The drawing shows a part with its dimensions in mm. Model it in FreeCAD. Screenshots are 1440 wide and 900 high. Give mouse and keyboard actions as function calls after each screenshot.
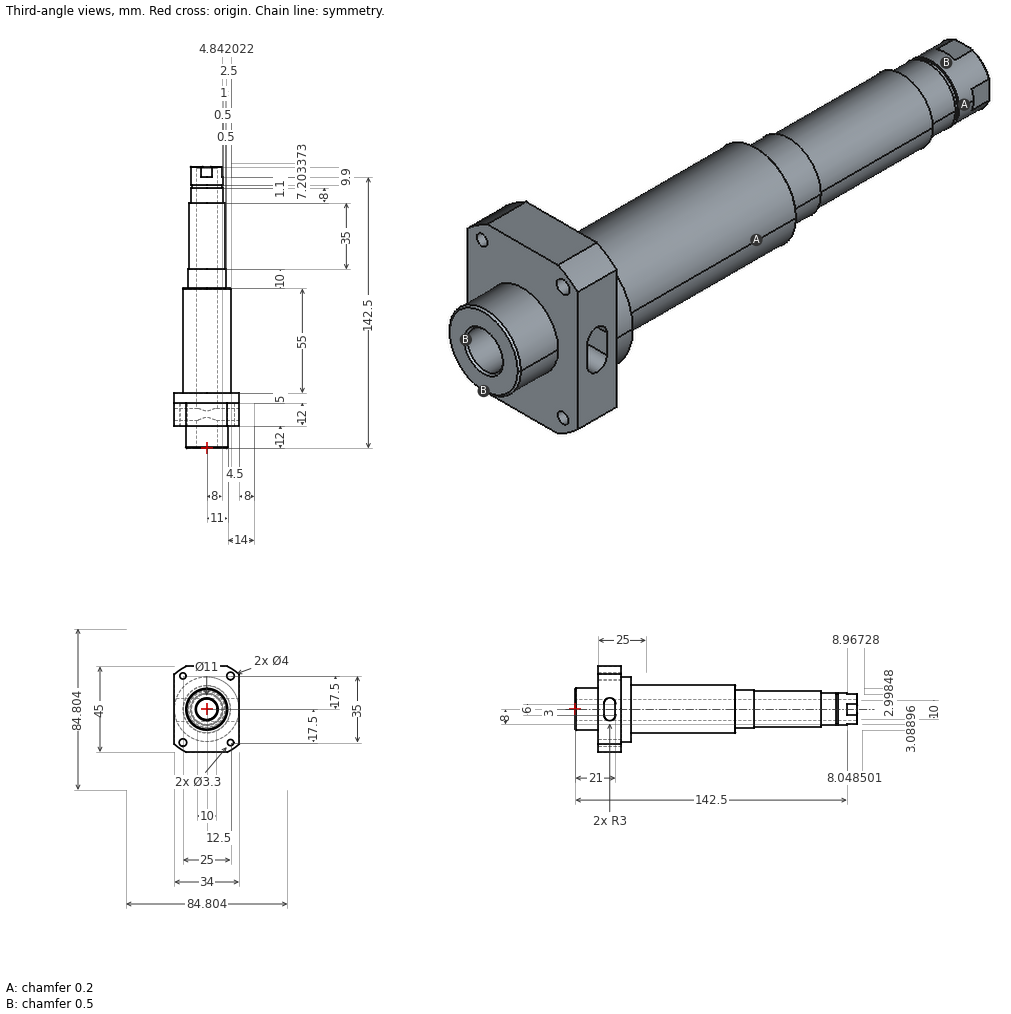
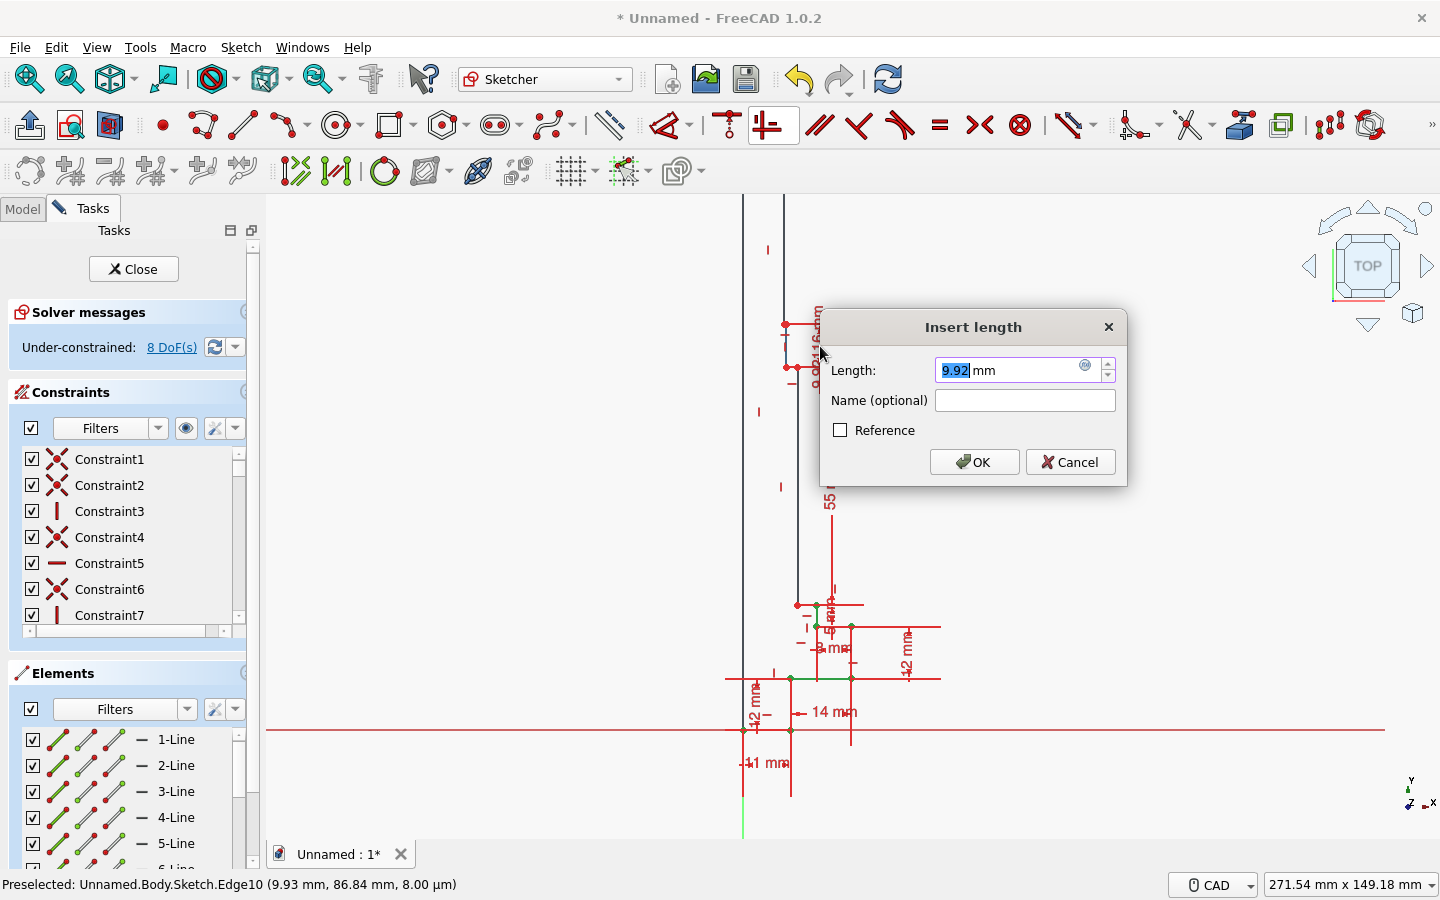
text(10)
key(Return)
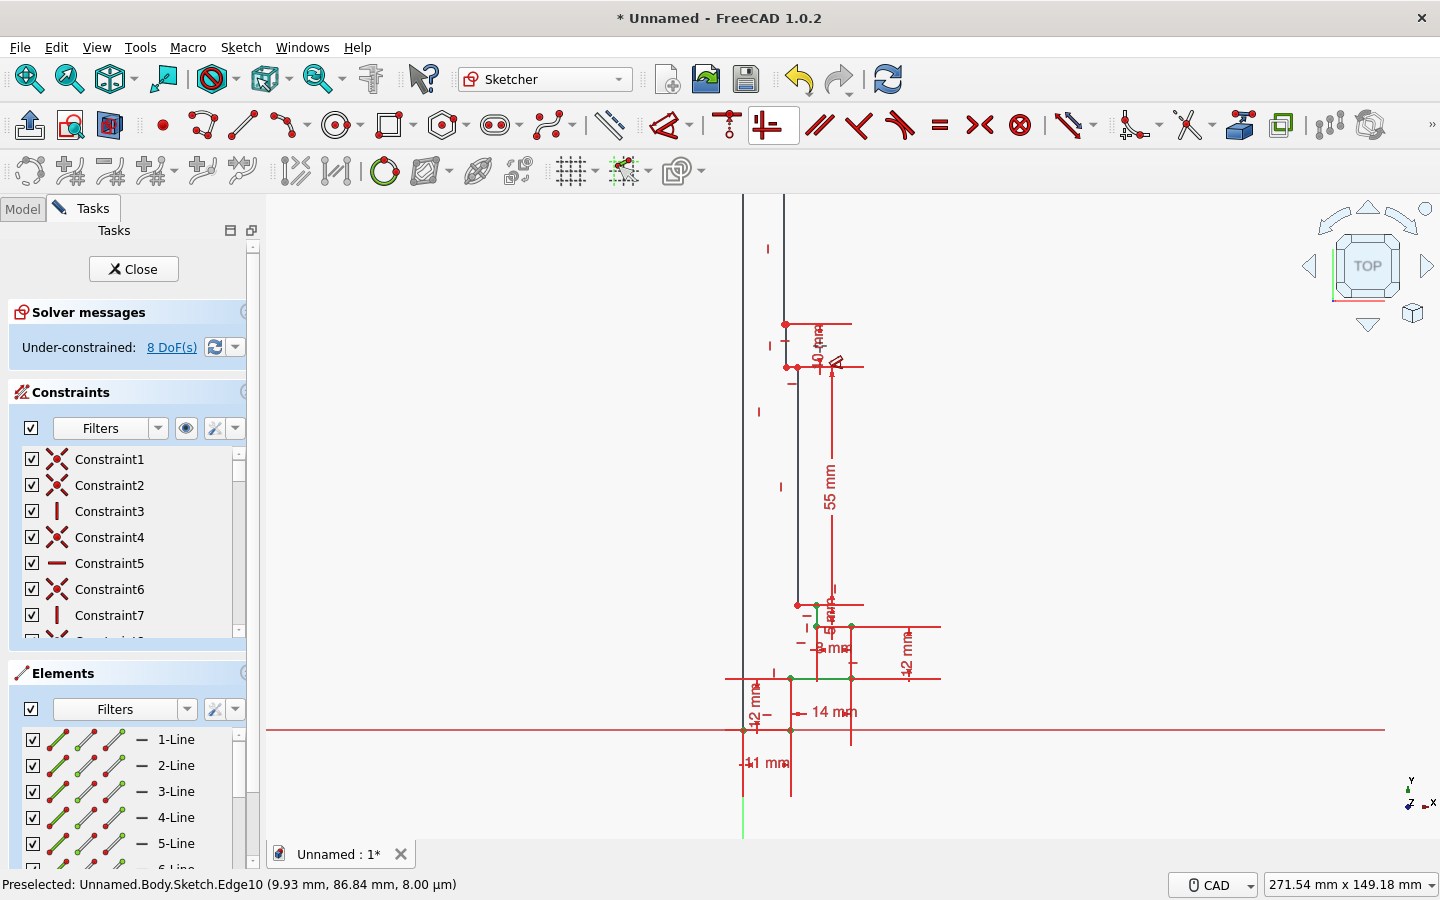
click(784, 279)
click(818, 273)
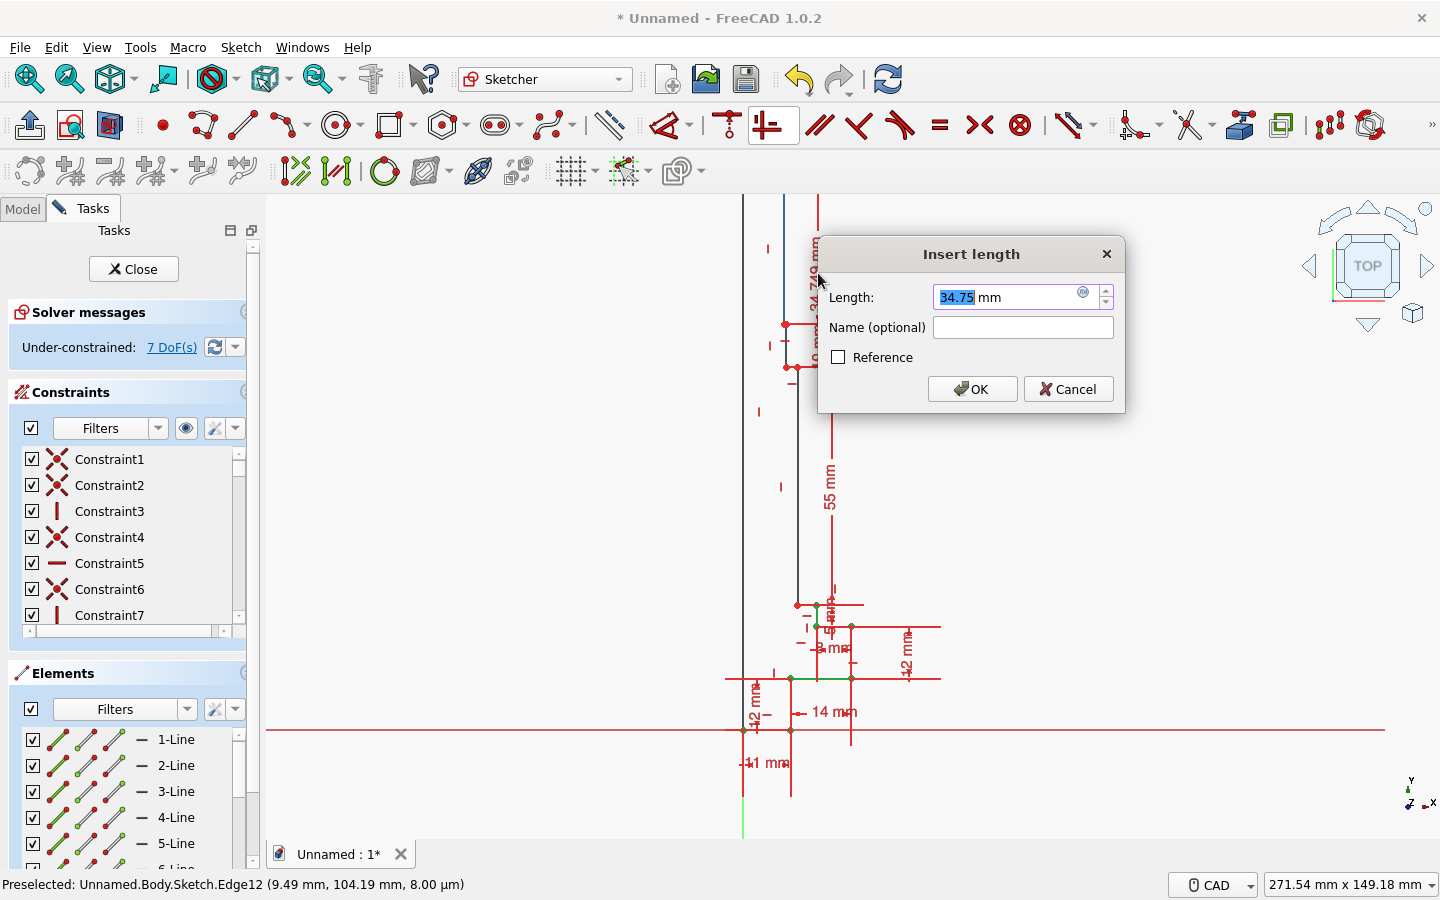
text(35)
key(Return)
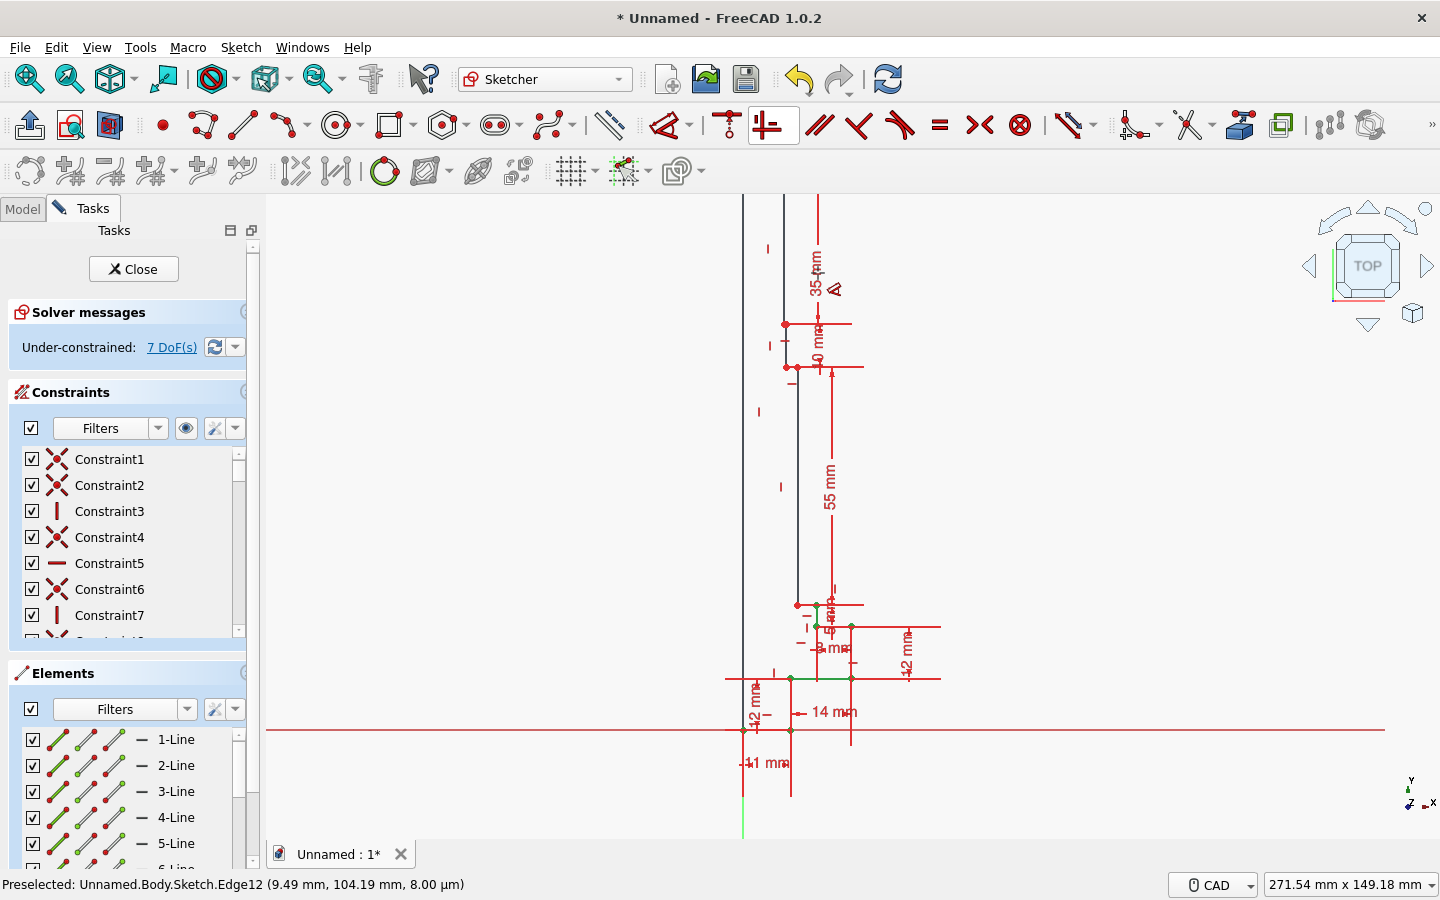
scroll(758, 732, down, 2)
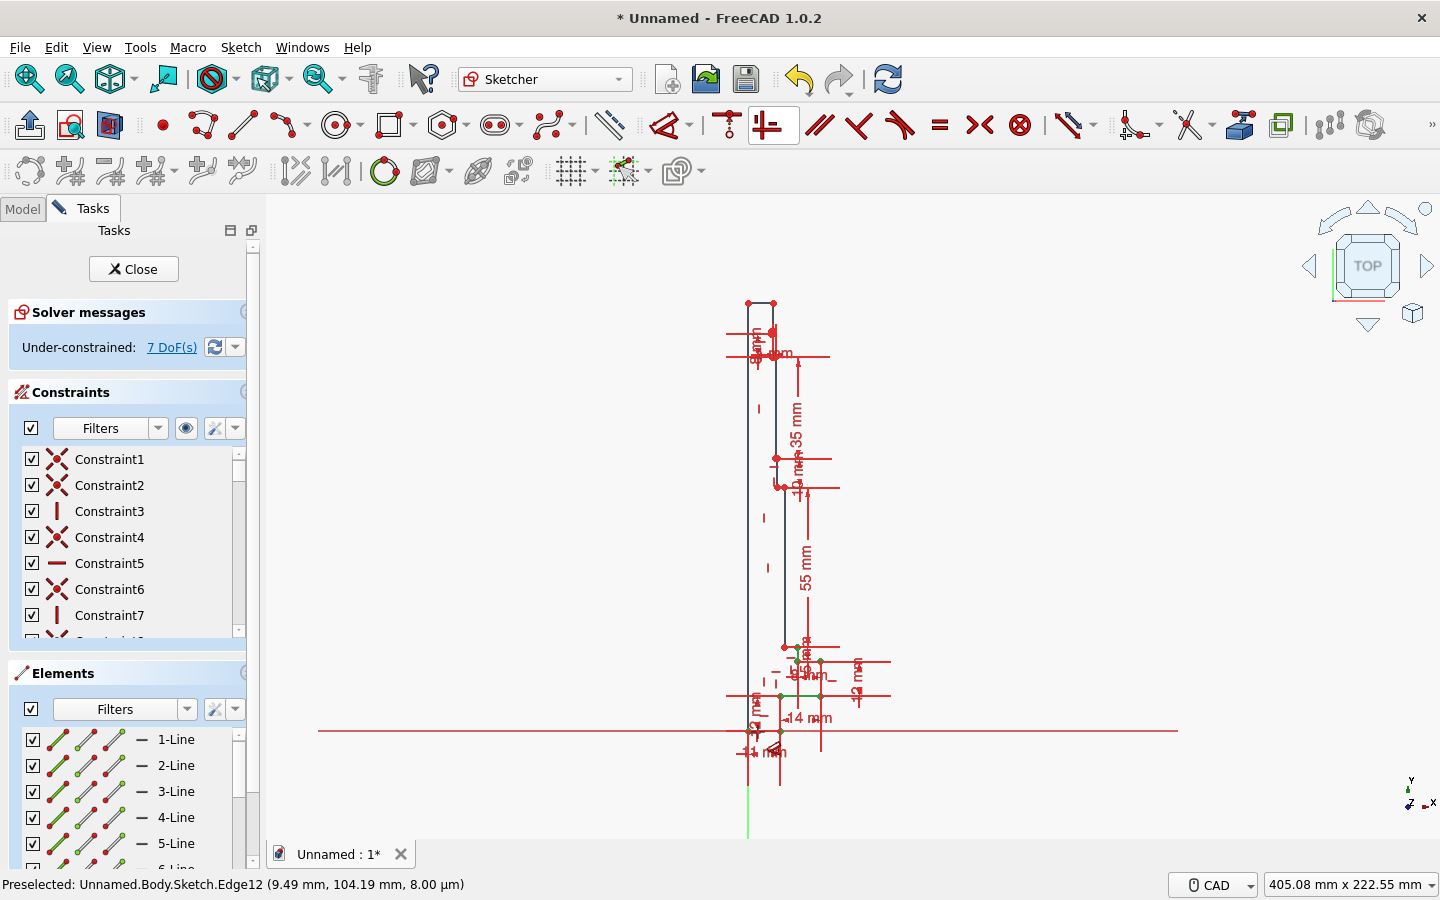
scroll(772, 334, up, 11)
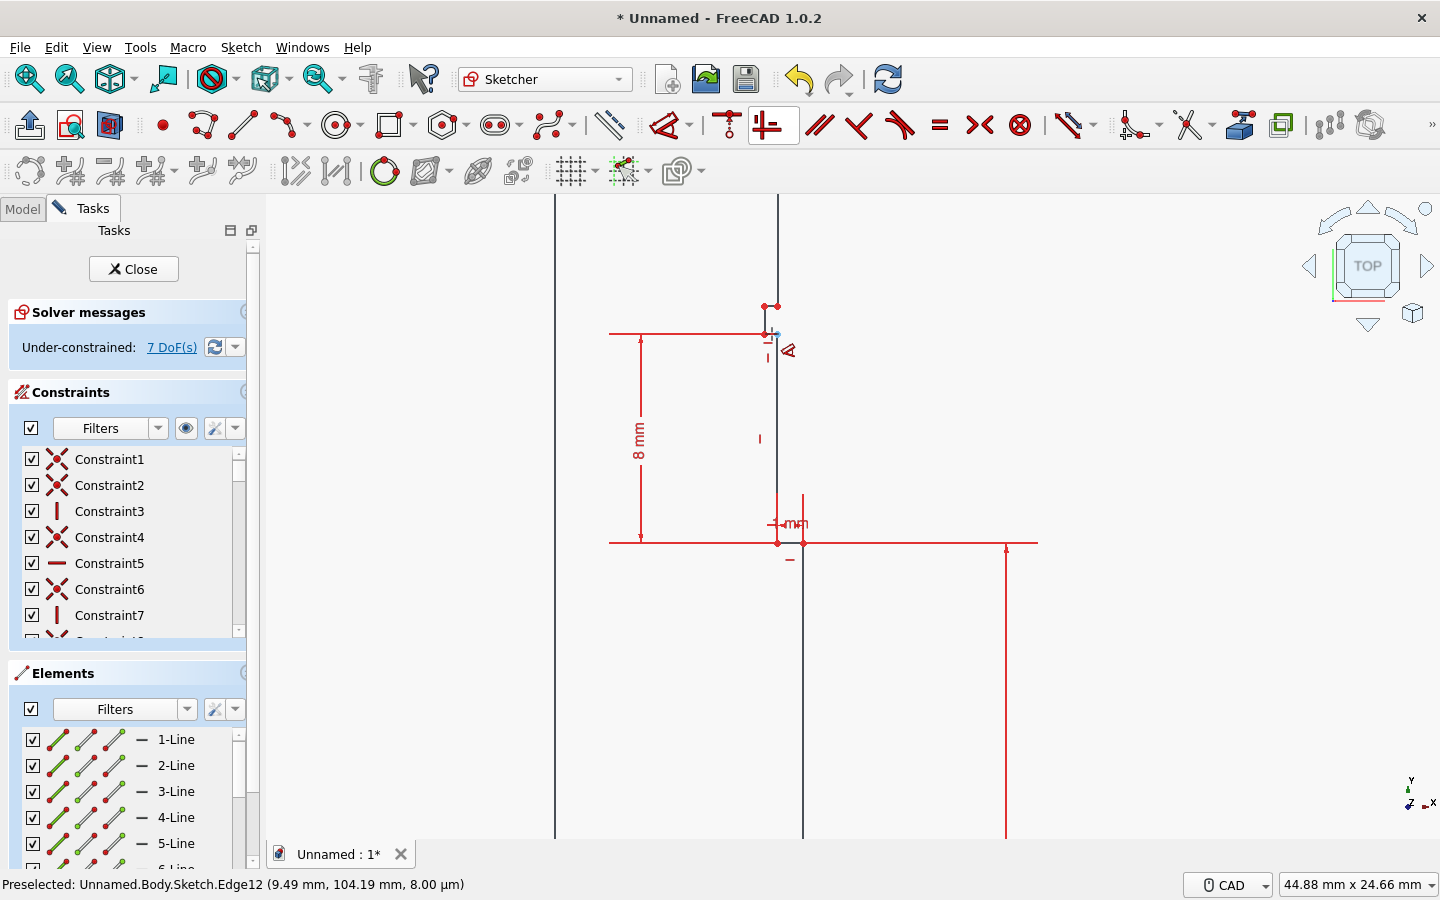
click(765, 334)
click(660, 300)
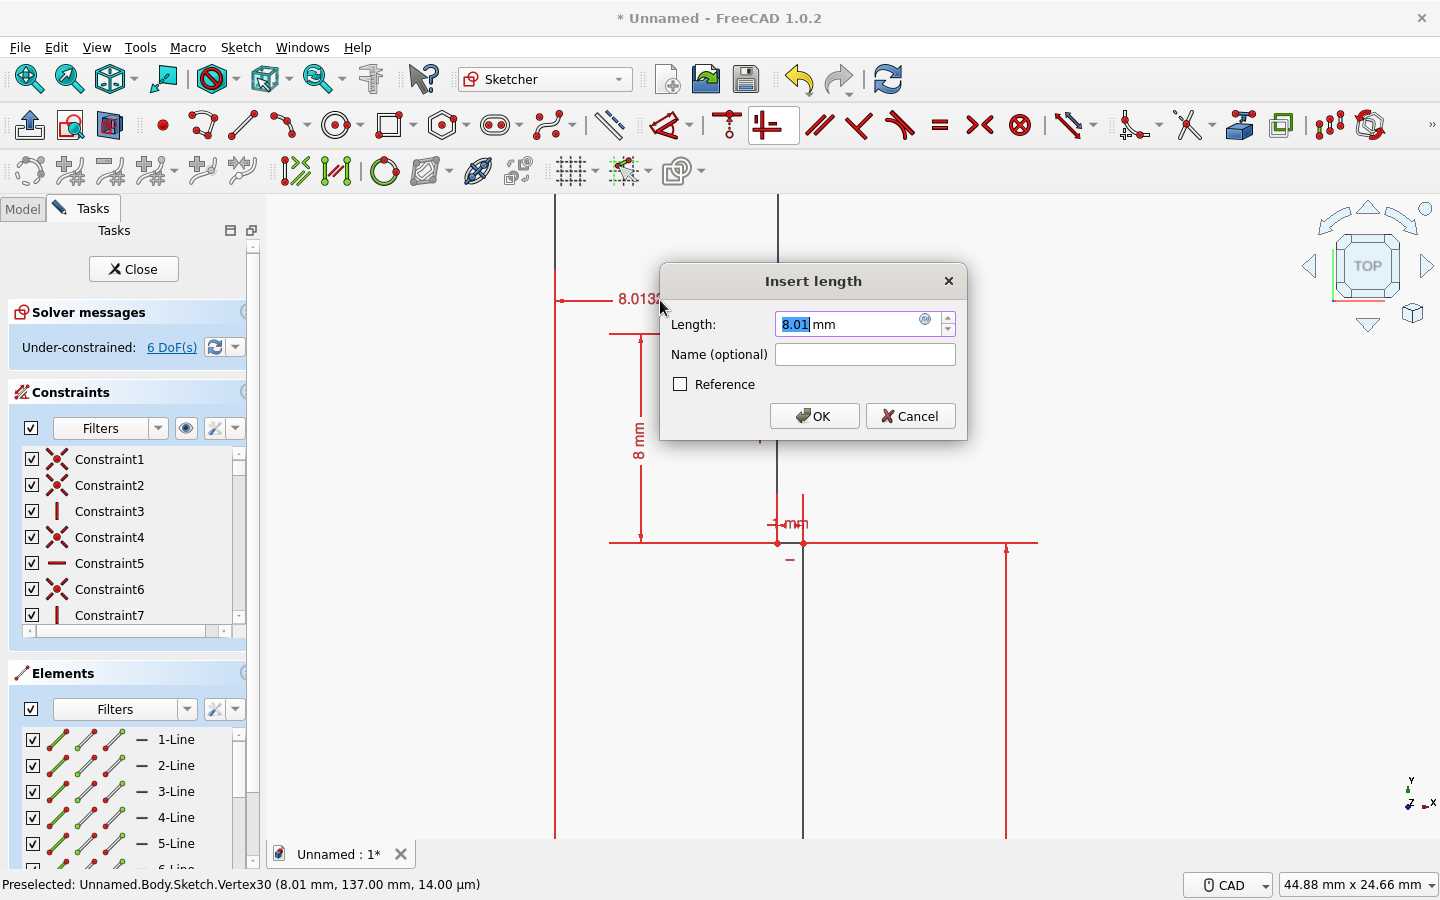
text(8)
key(Return)